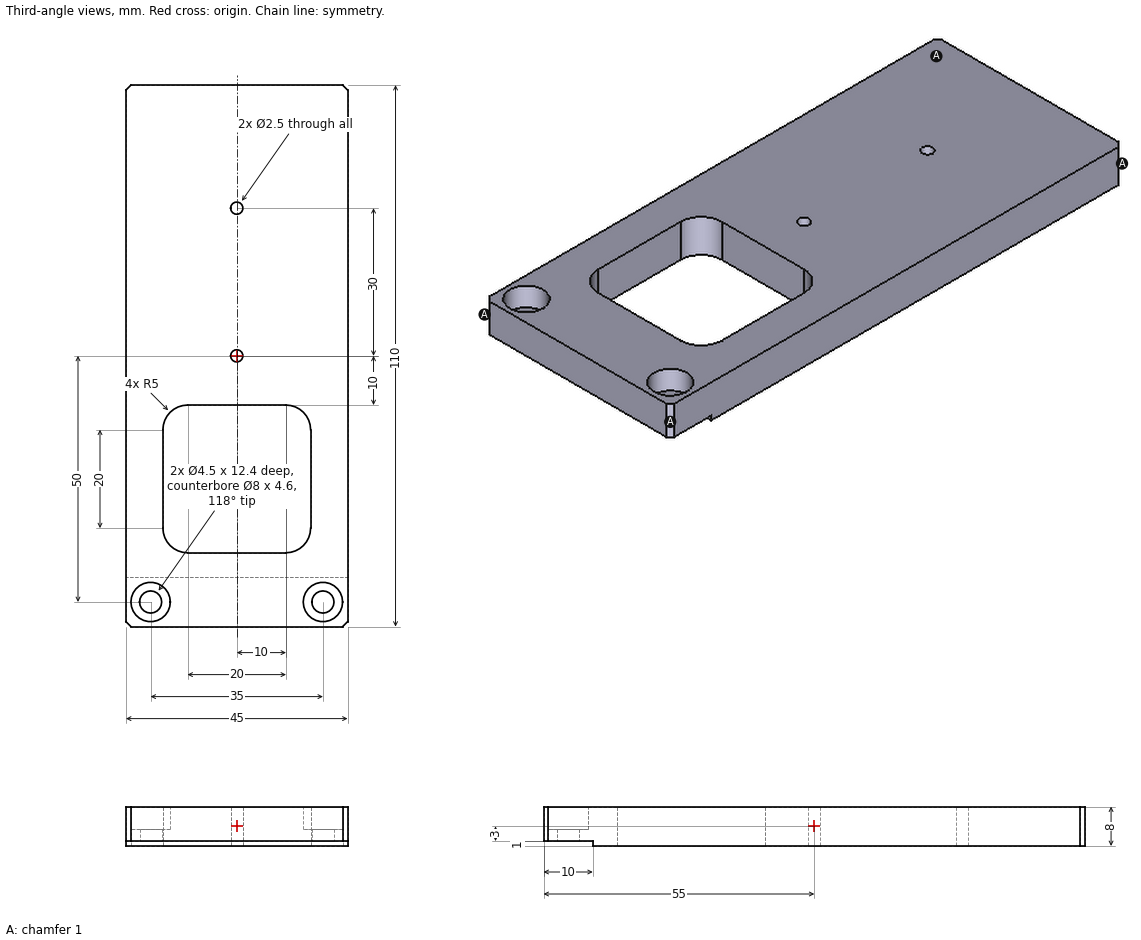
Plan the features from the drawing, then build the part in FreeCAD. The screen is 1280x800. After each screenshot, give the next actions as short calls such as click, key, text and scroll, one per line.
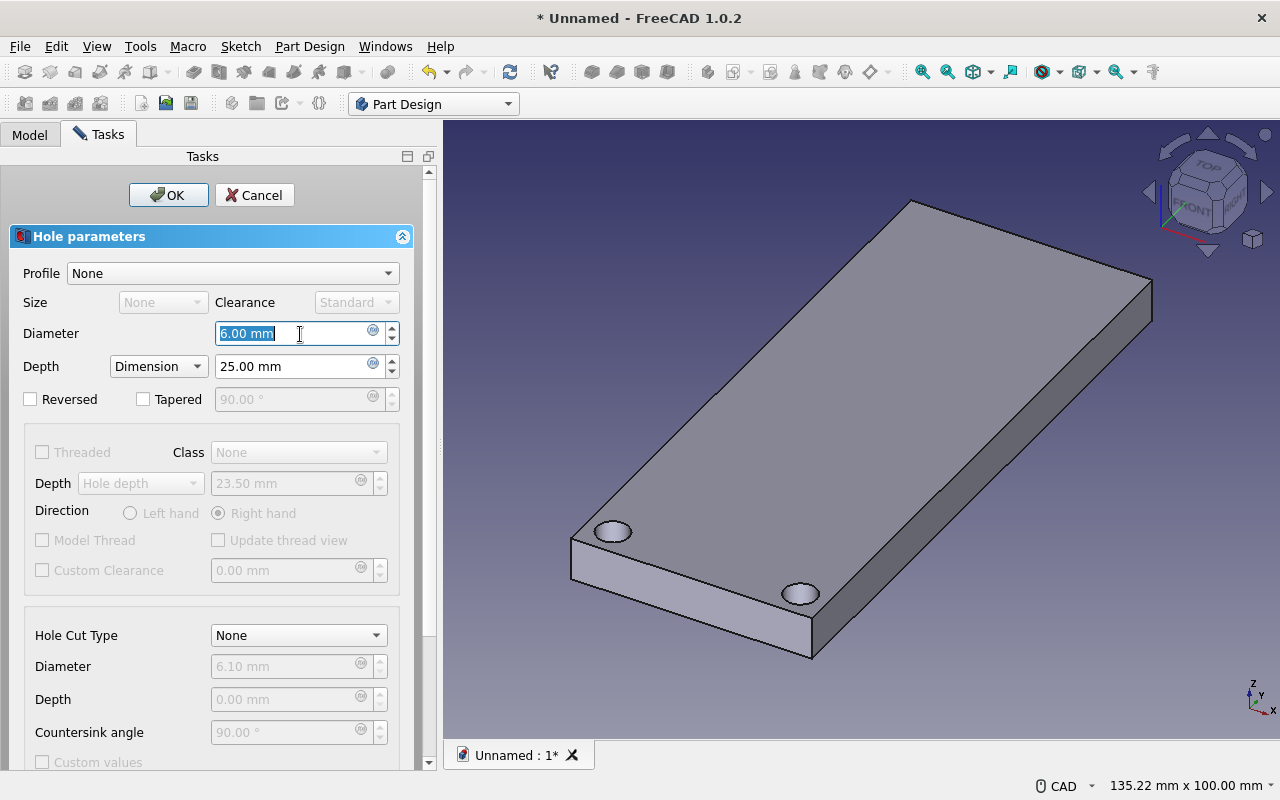
text(4.5)
key(Tab)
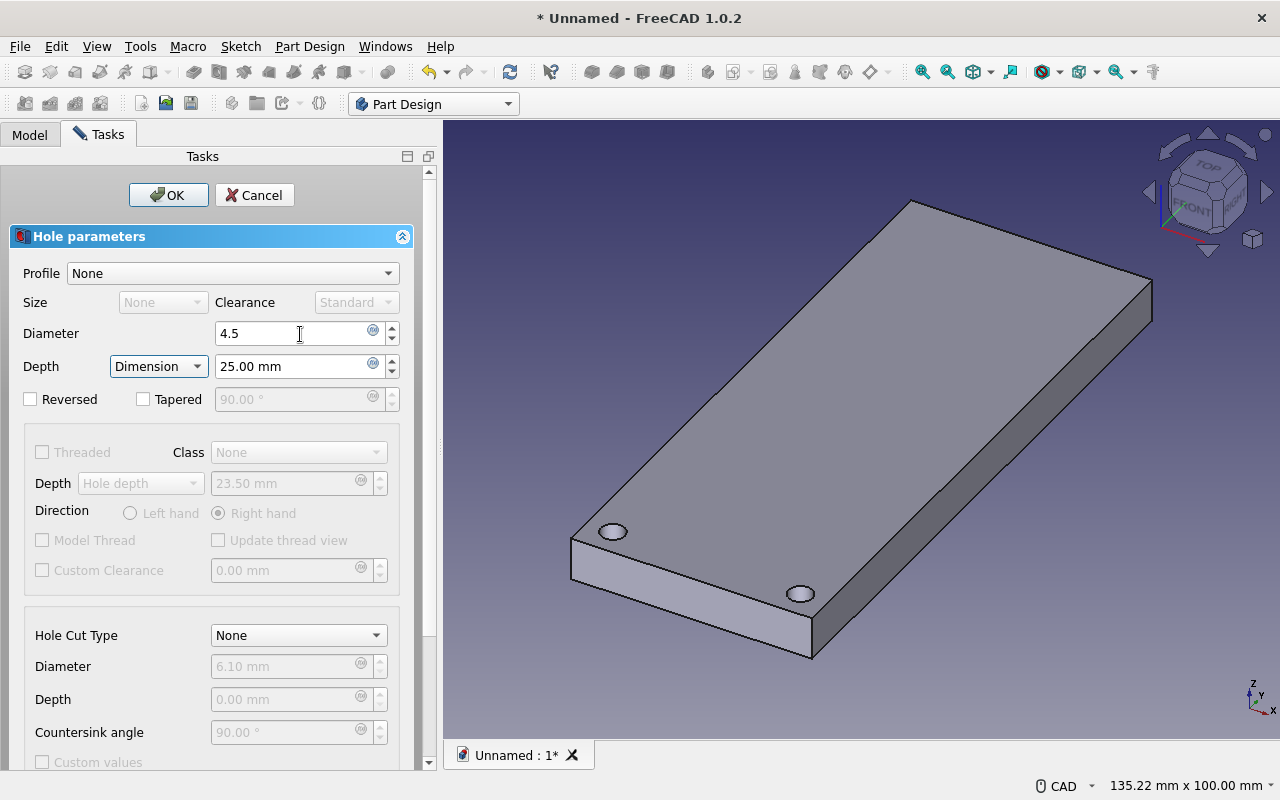
triple_click(300, 366)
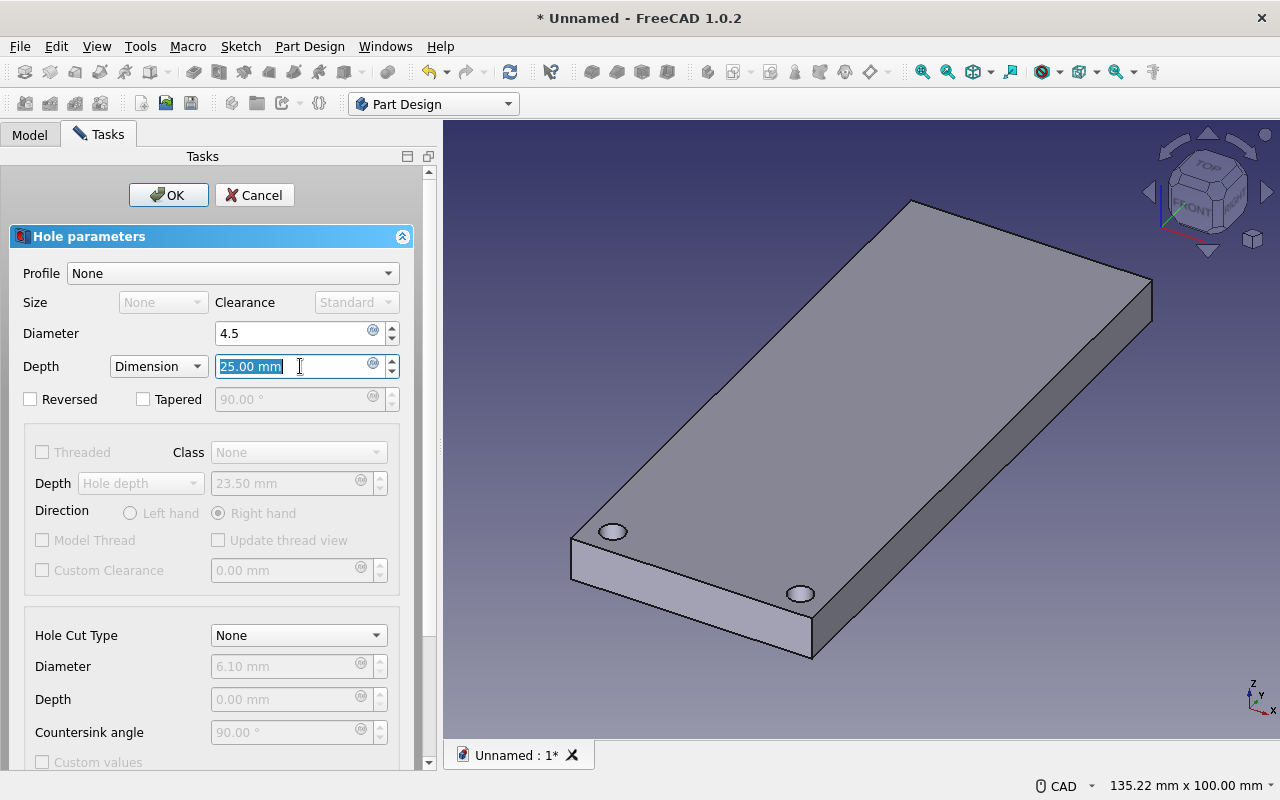
text(12.4)
key(Tab)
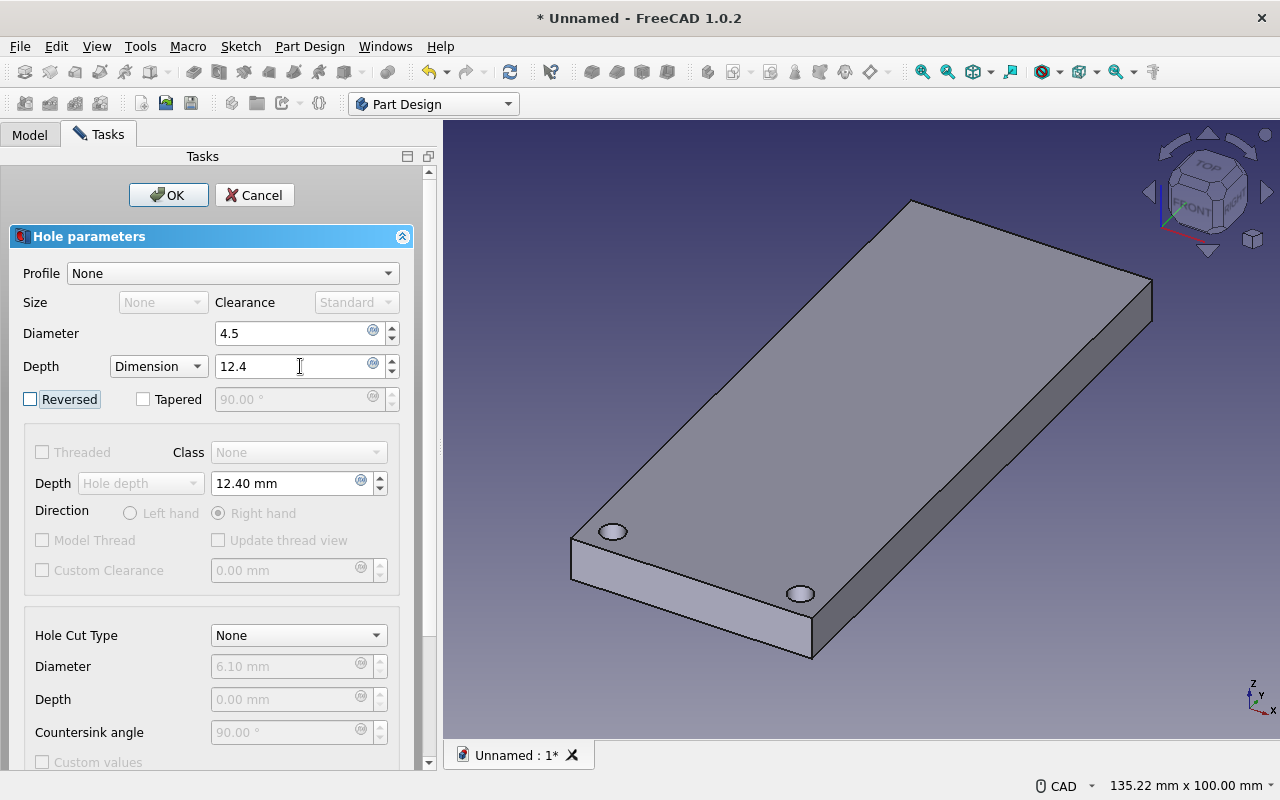
click(300, 636)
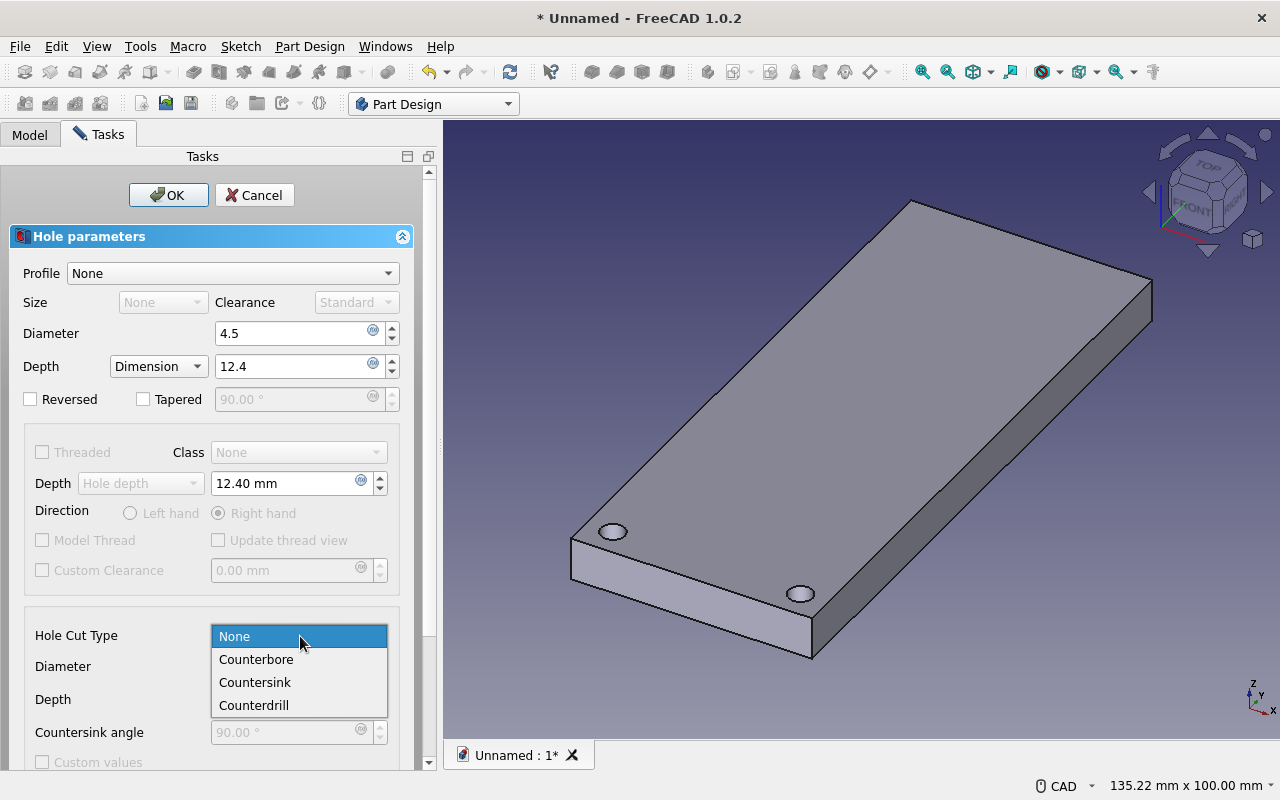
click(298, 660)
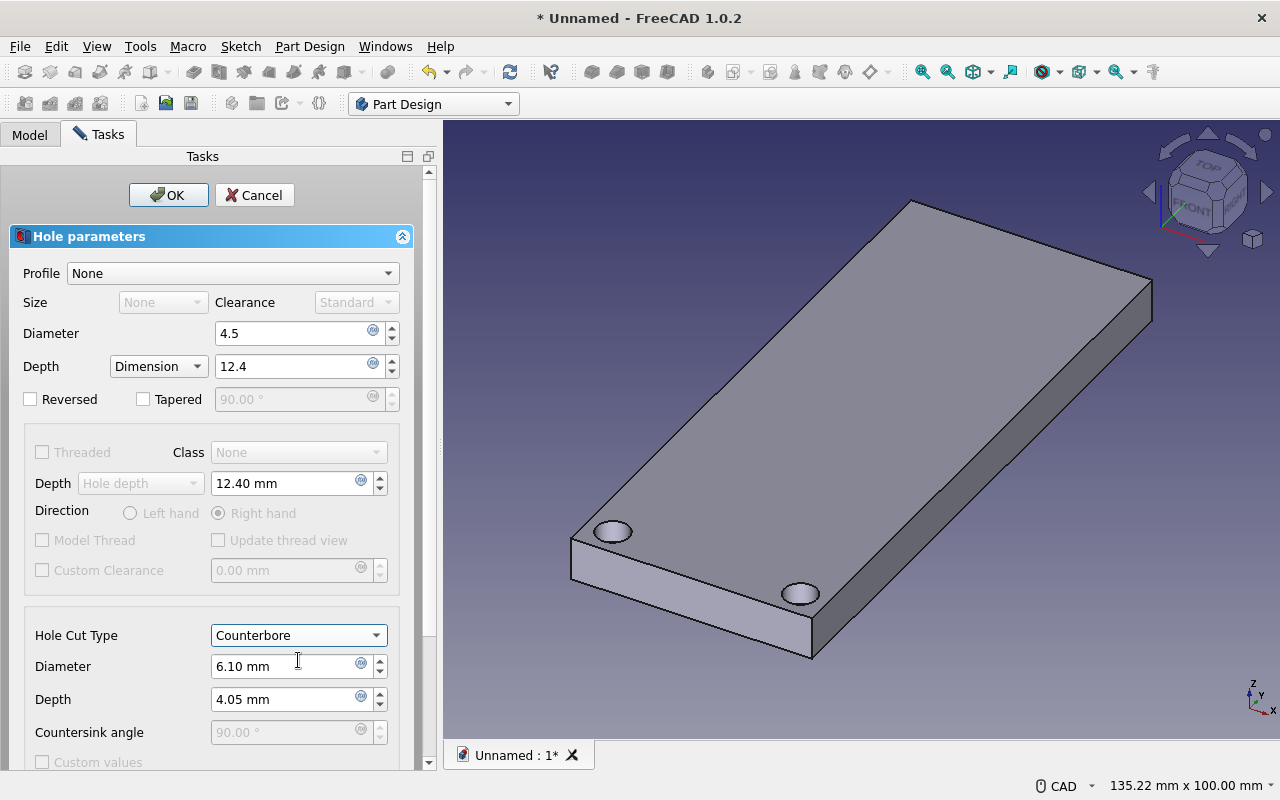
triple_click(292, 666)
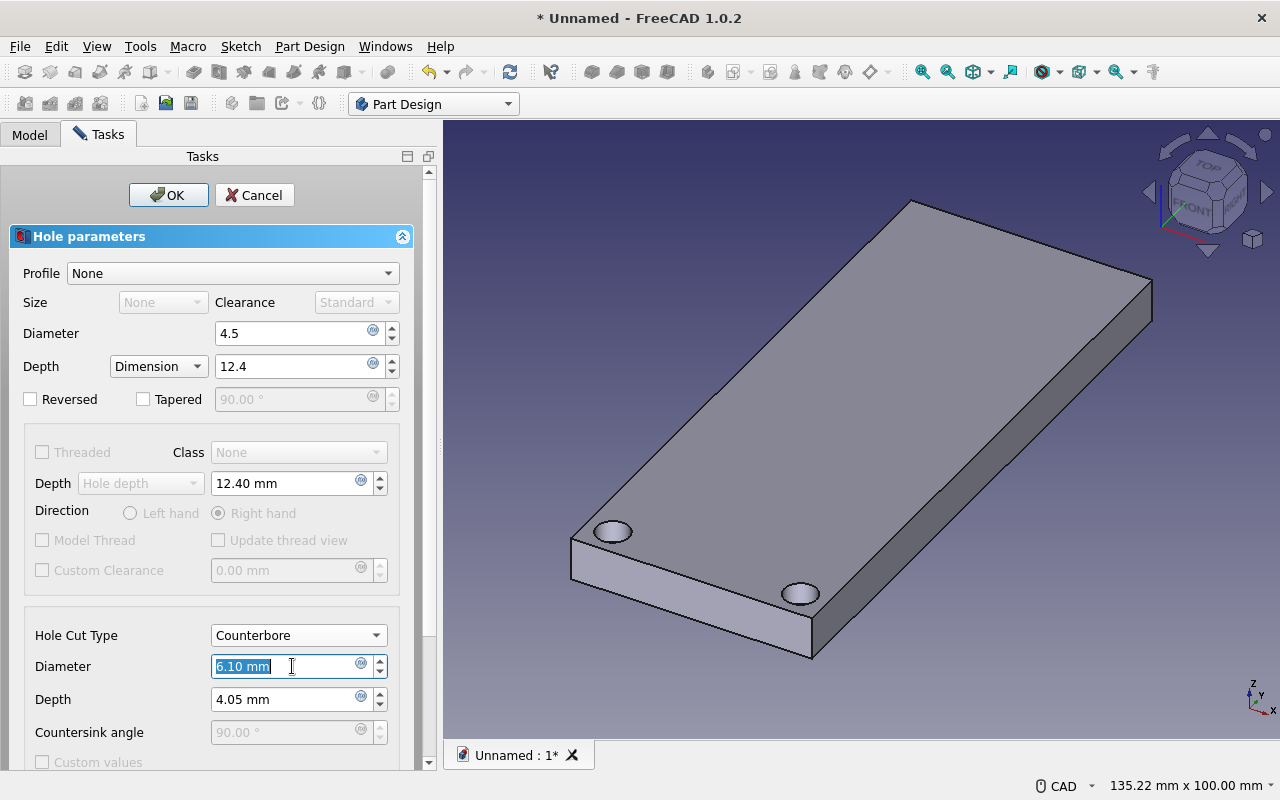
text(8)
key(Tab)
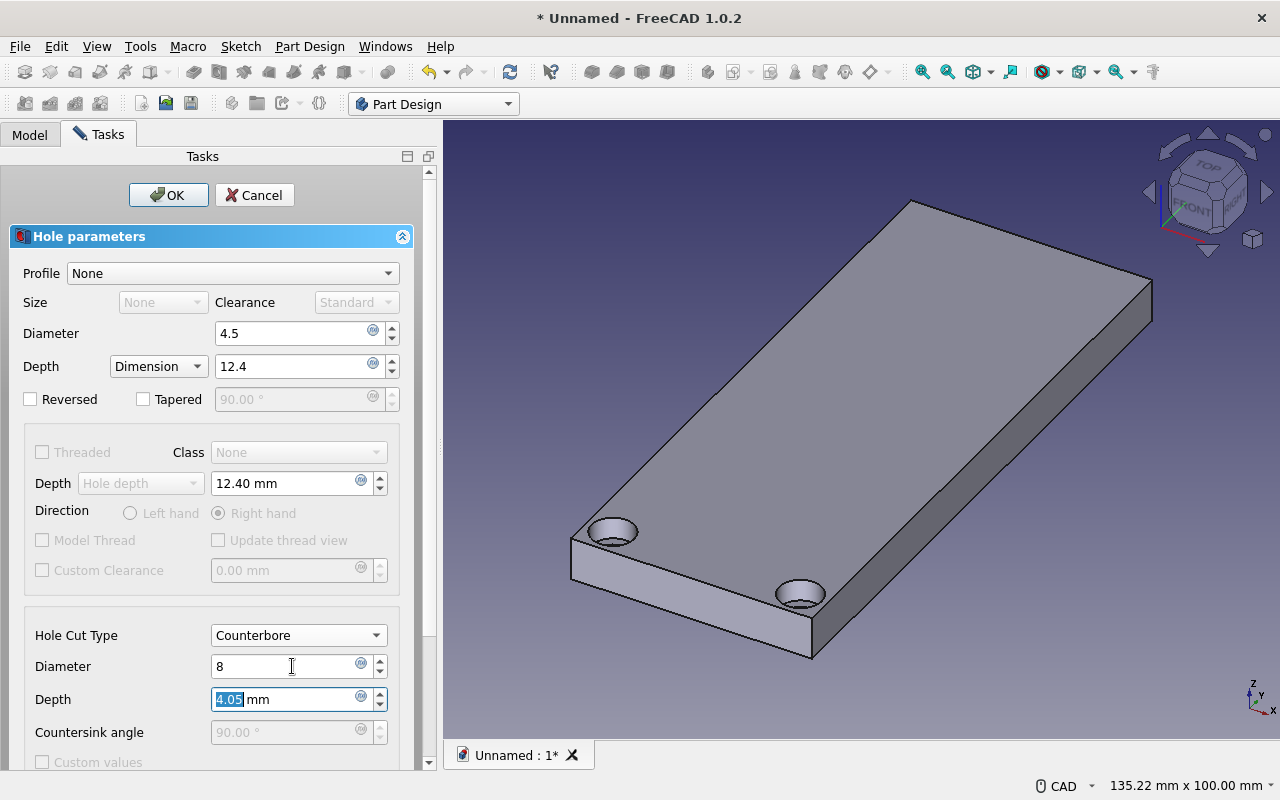
text(4.6)
key(Tab)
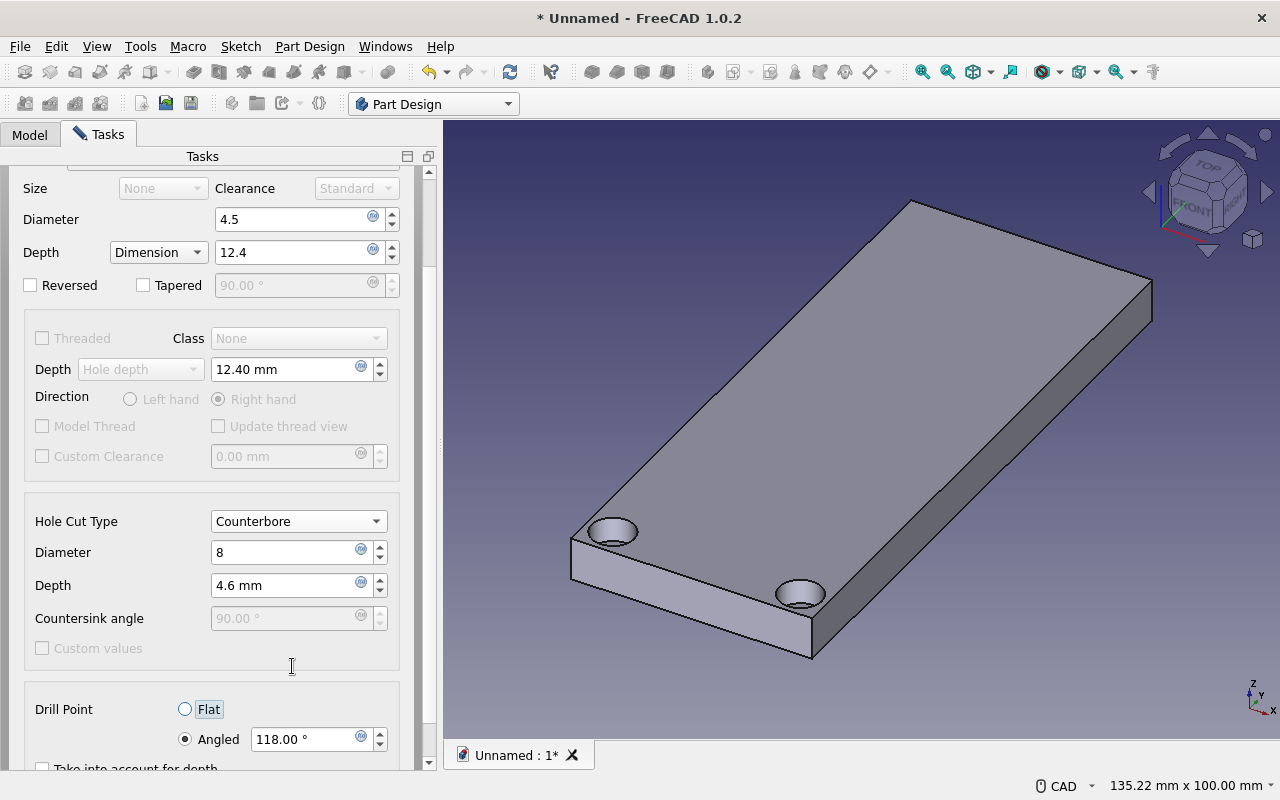
scroll(429, 468, up, 3)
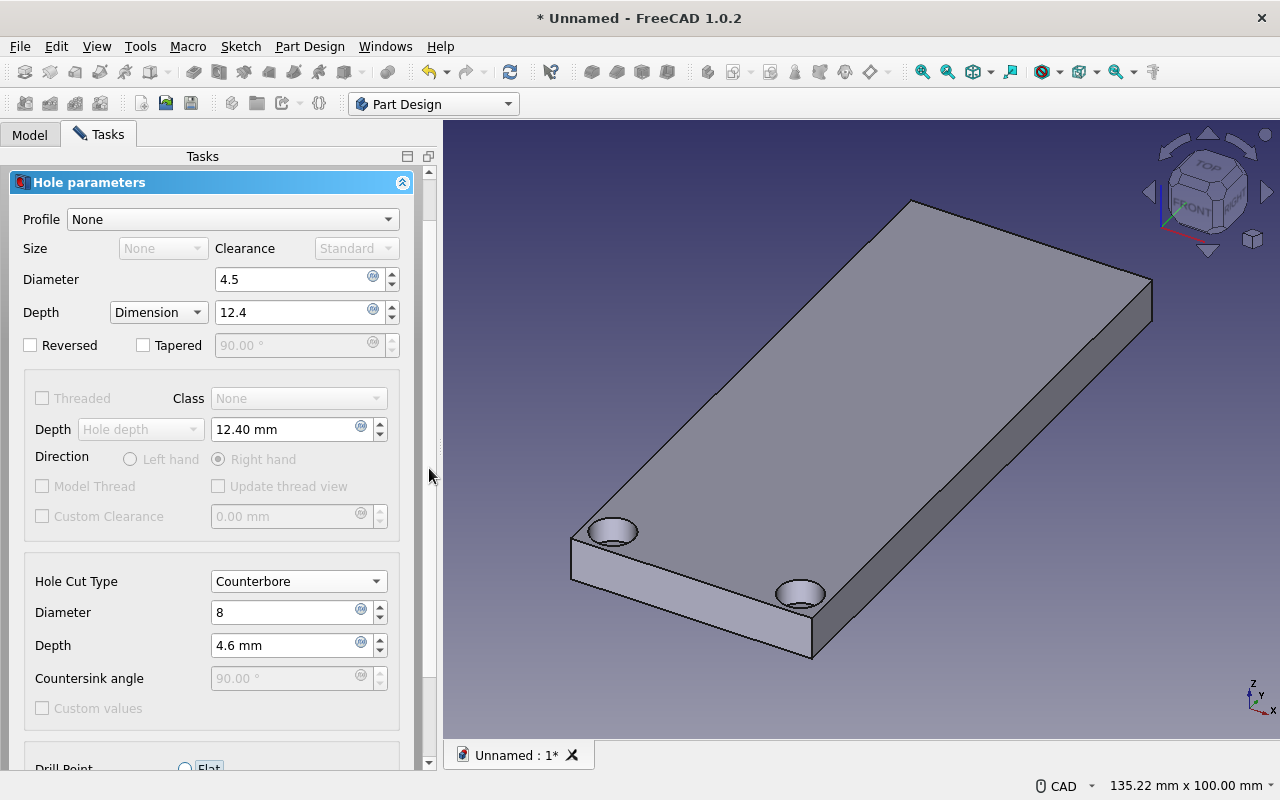
click(169, 195)